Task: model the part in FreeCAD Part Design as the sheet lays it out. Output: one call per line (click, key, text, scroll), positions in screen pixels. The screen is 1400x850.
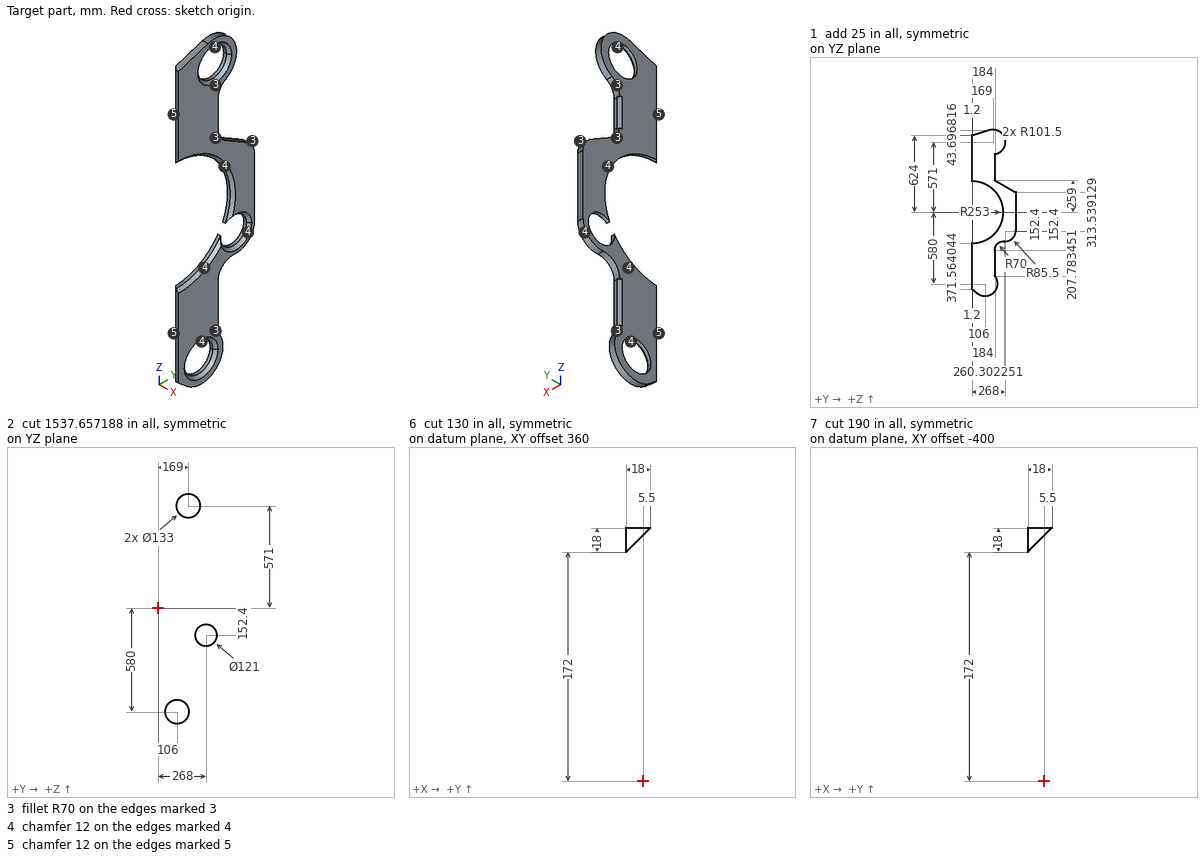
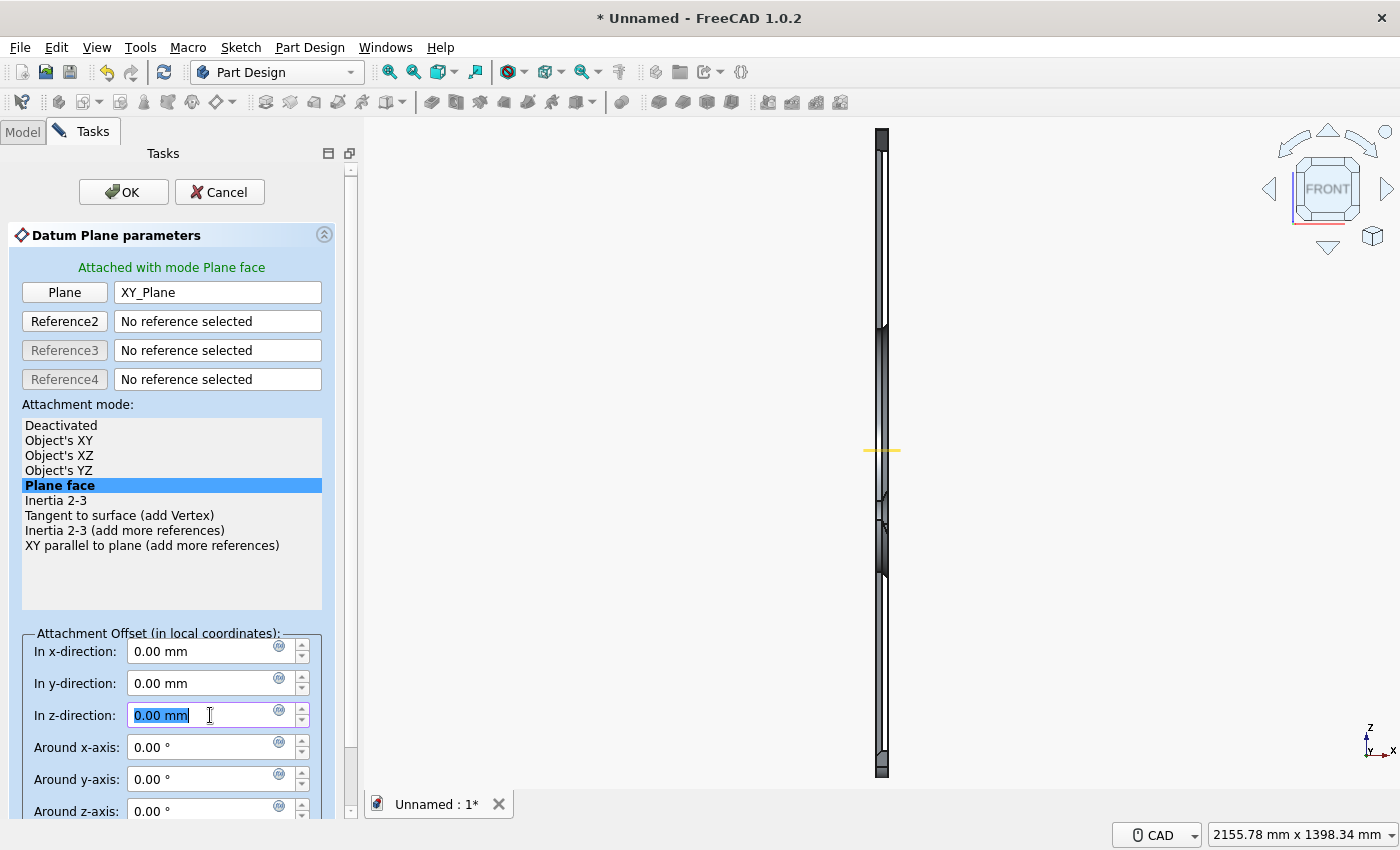
text(-400)
key(Tab)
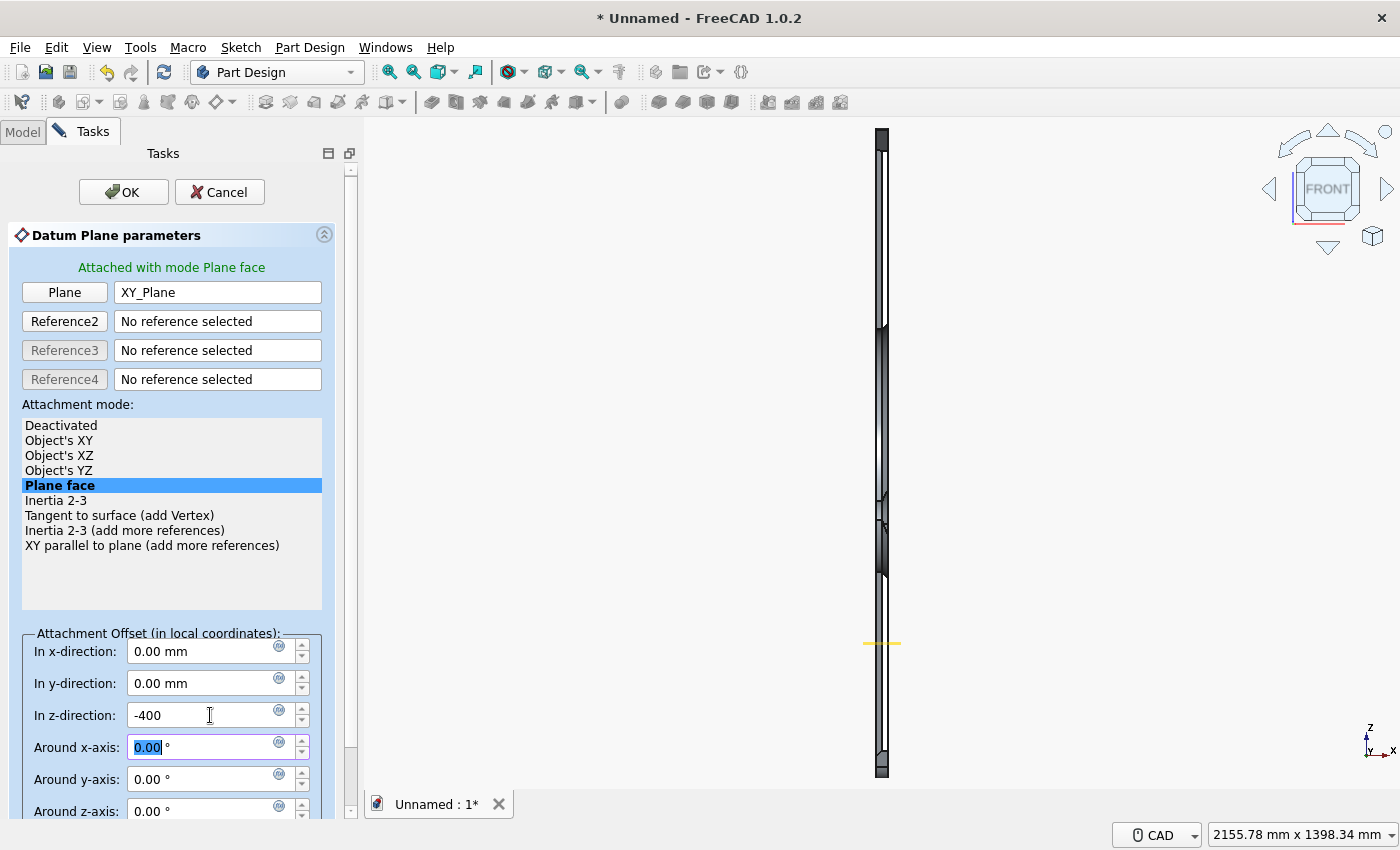
click(124, 192)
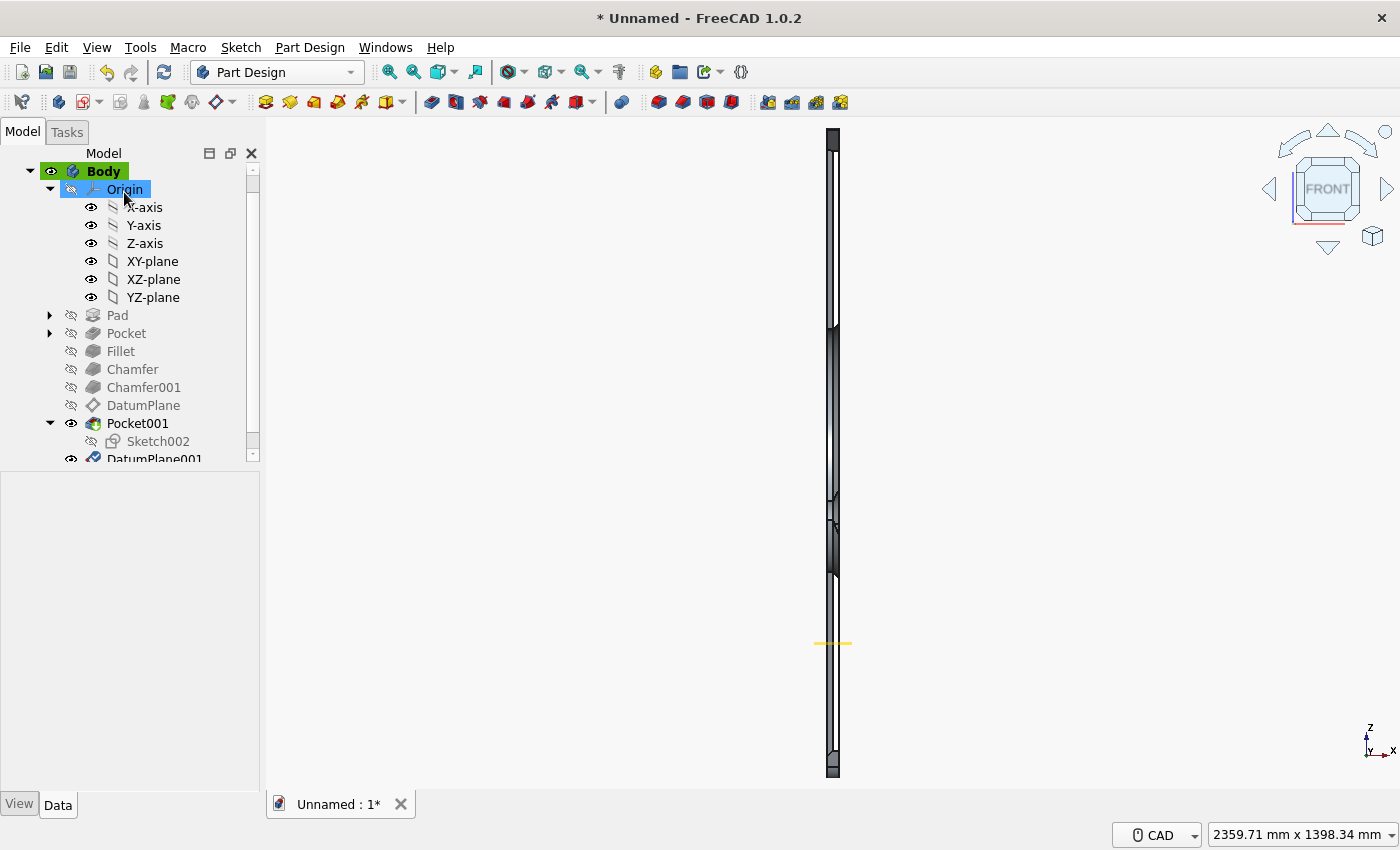
click(116, 459)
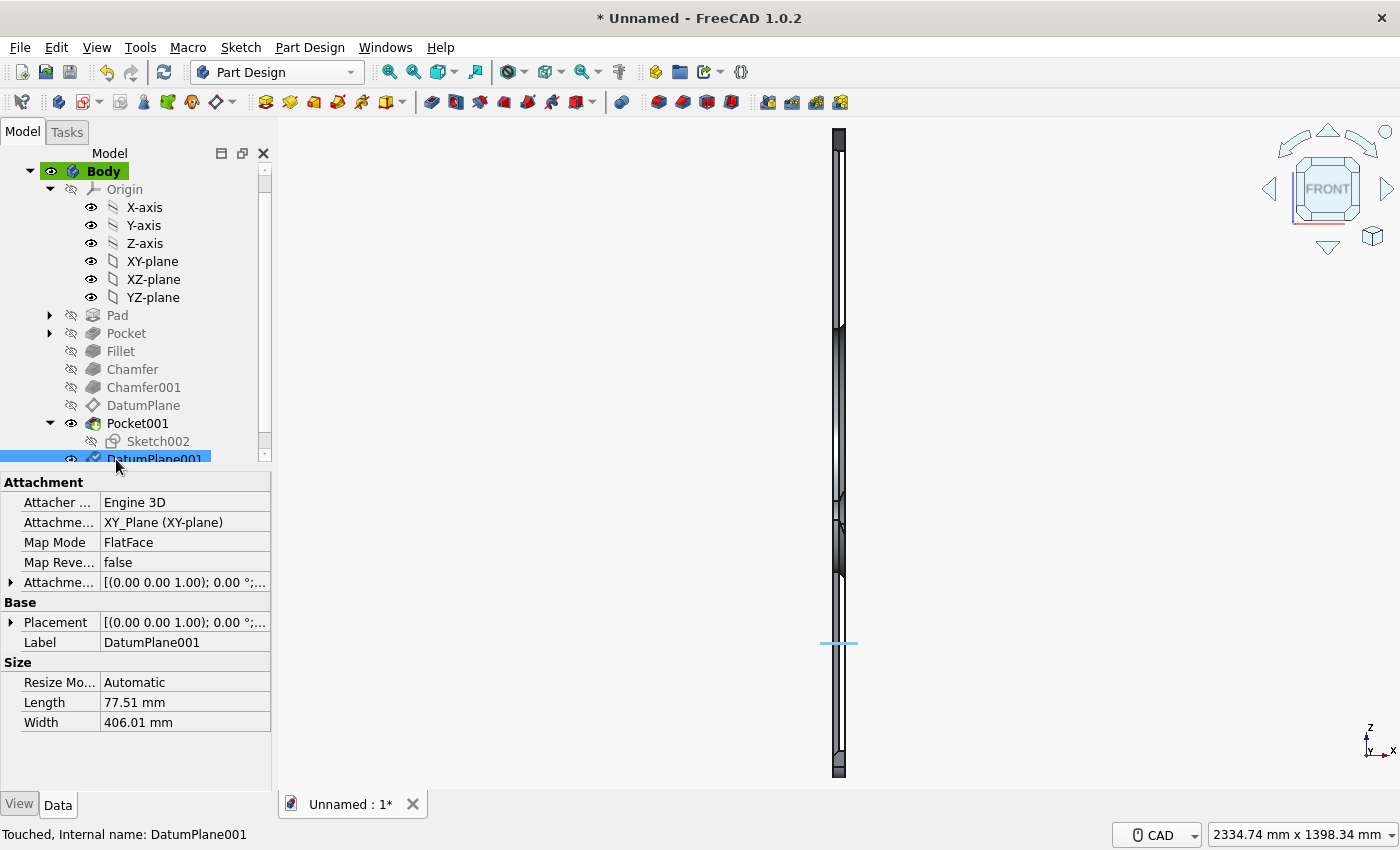
click(84, 102)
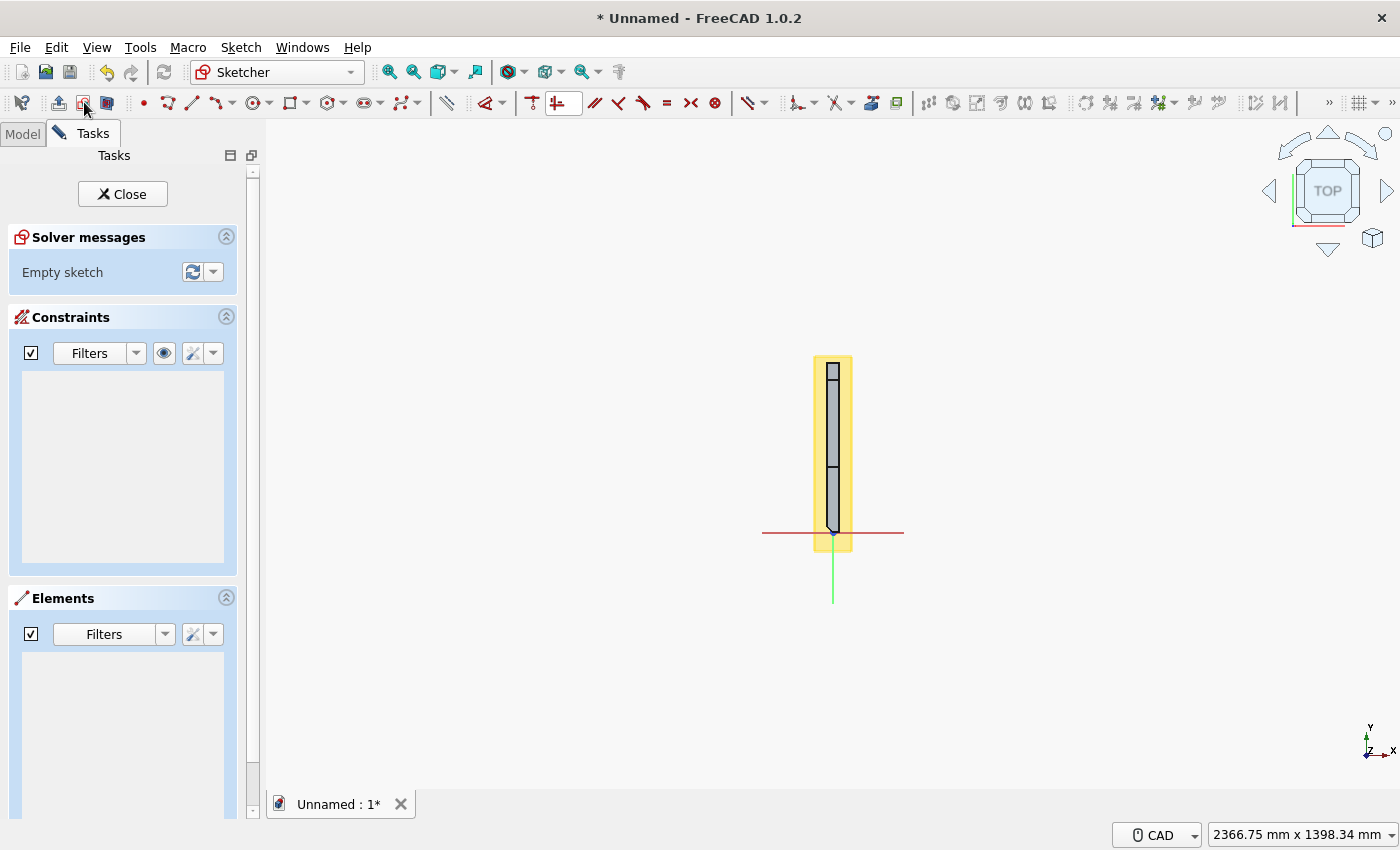
key(q)
key(s)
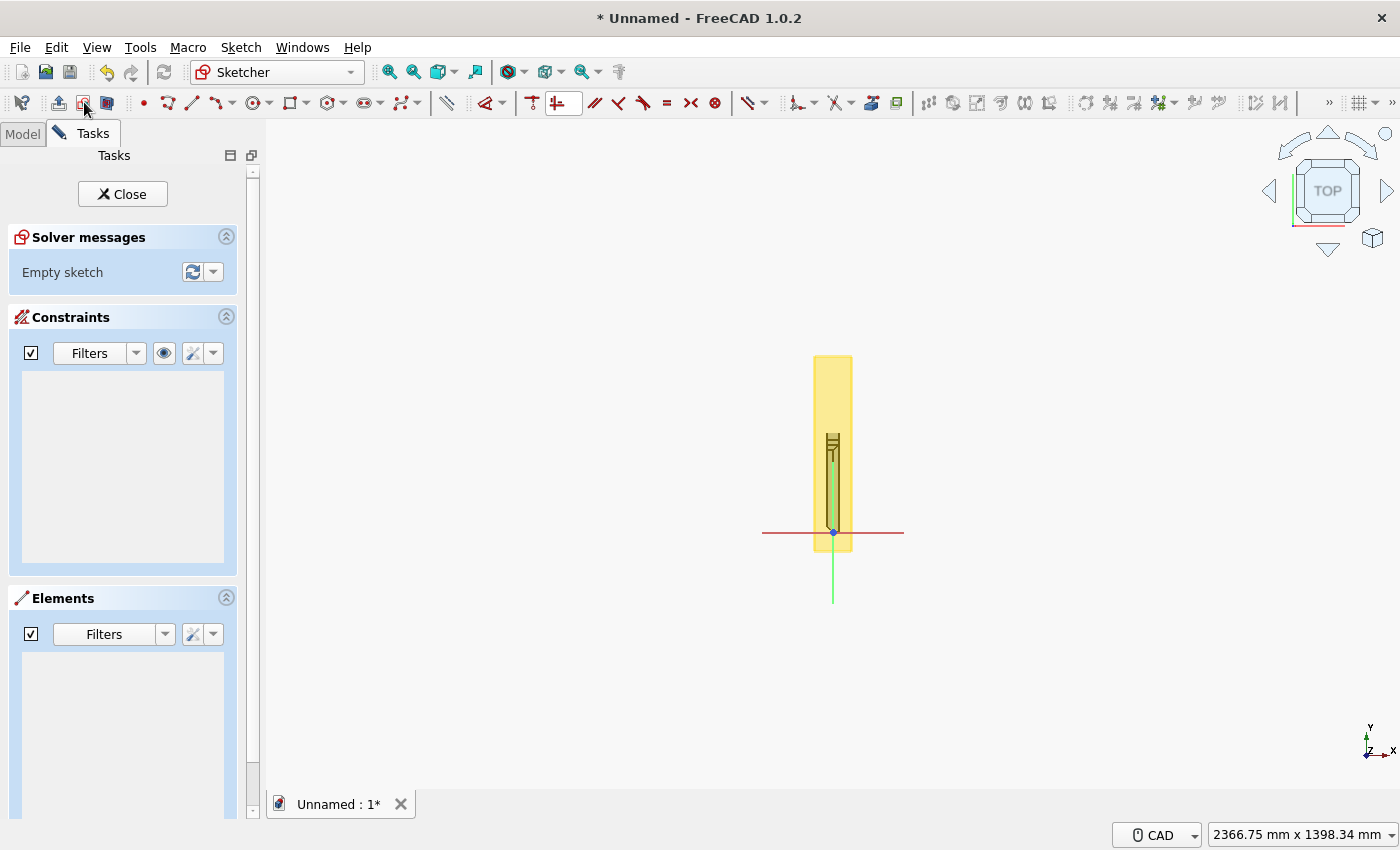
scroll(835, 446, up, 15)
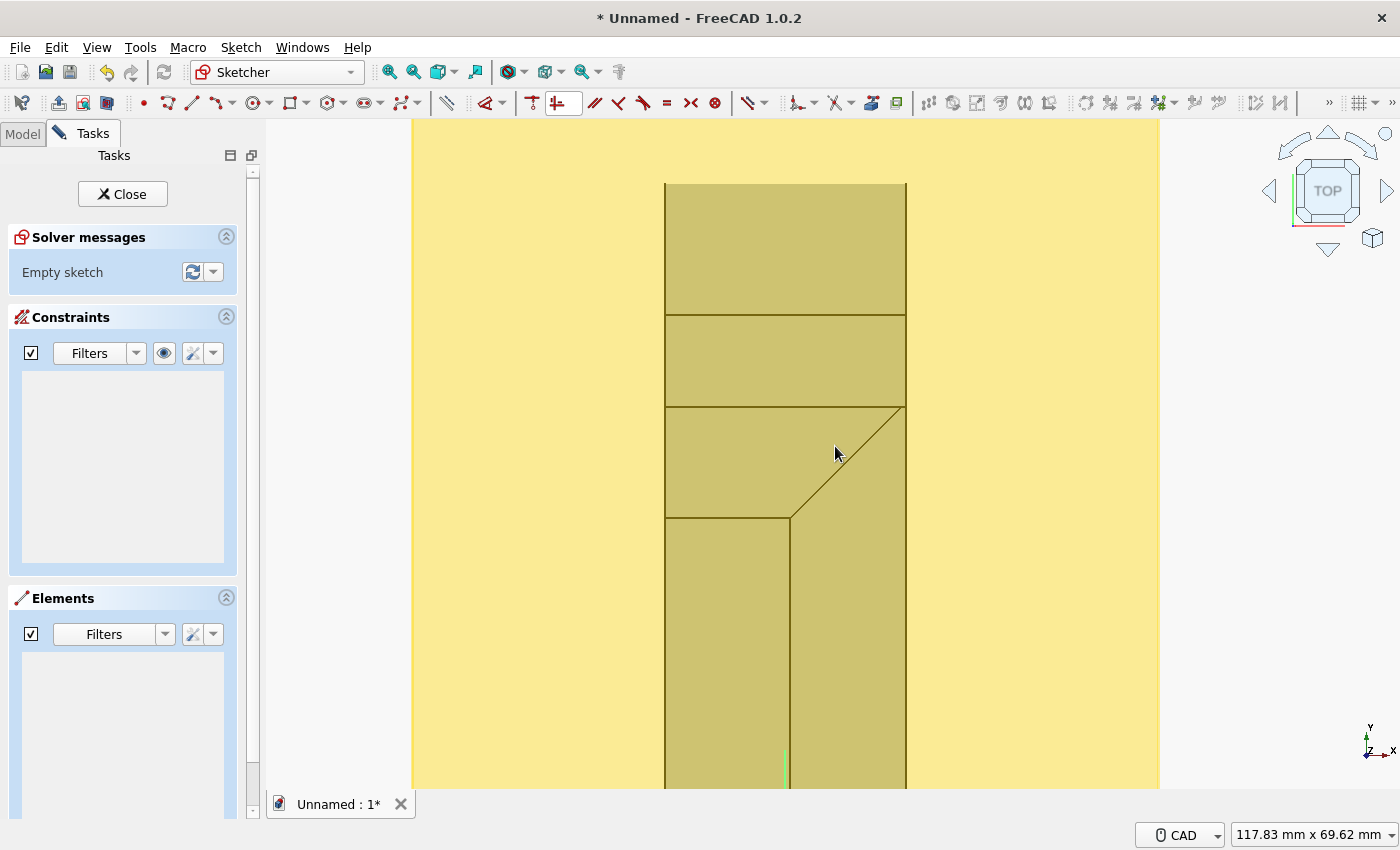
scroll(744, 426, up, 5)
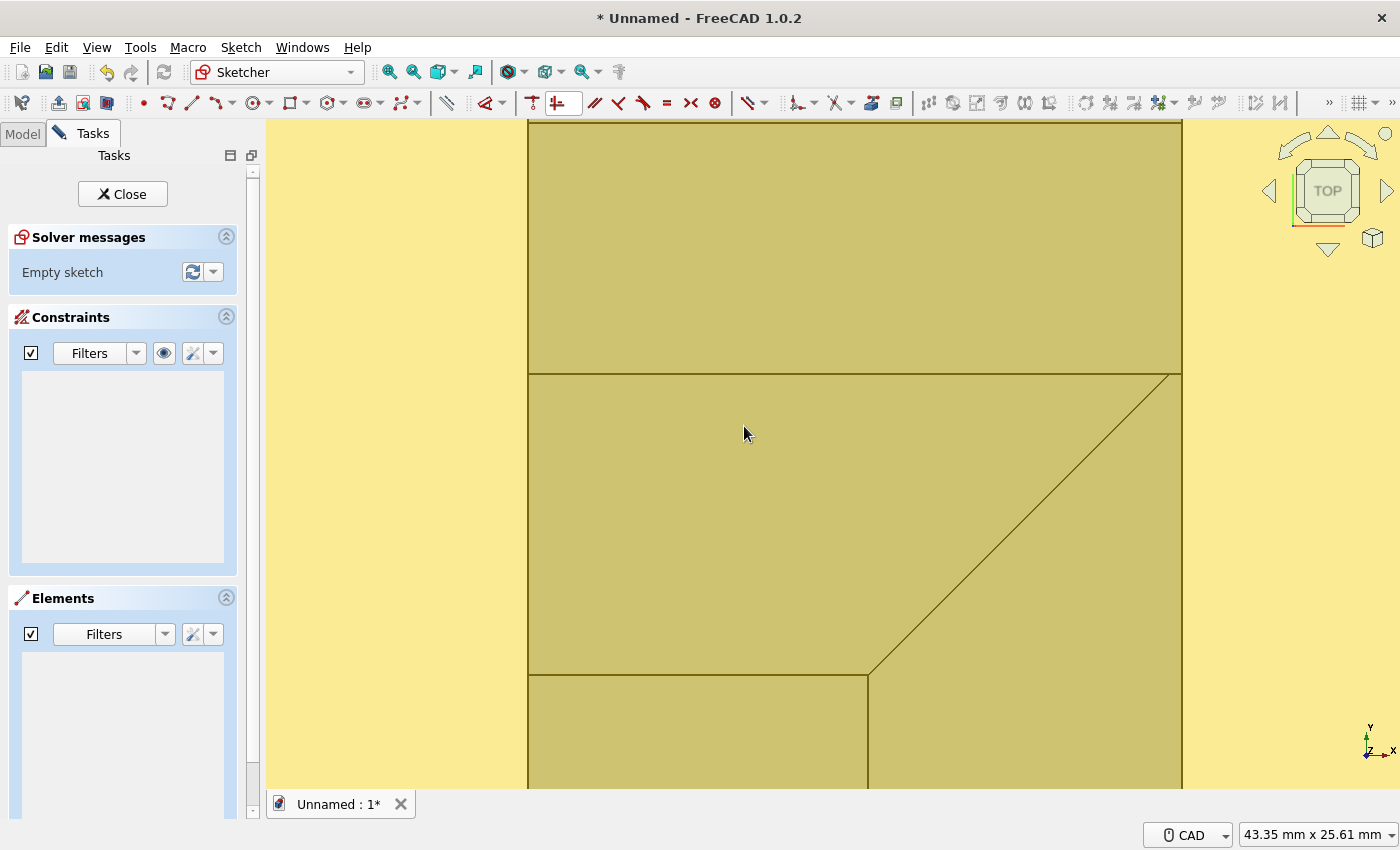
click(168, 104)